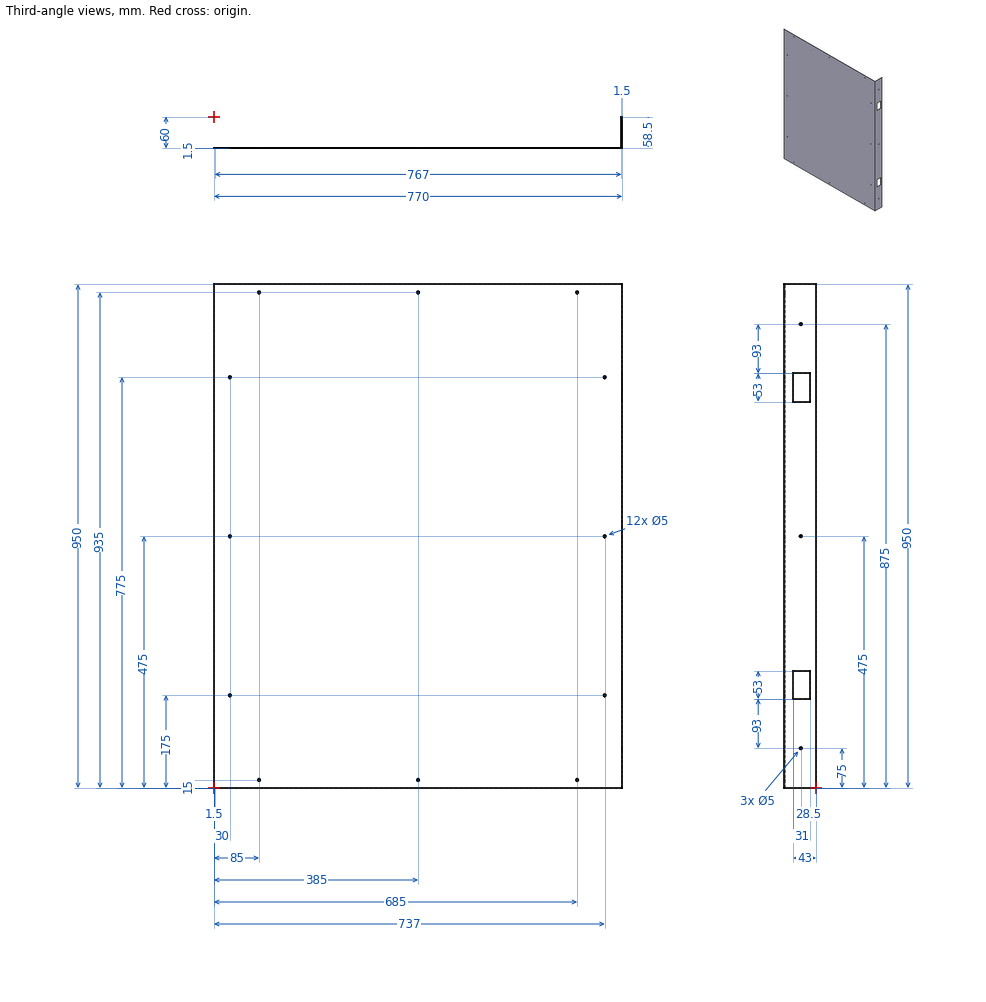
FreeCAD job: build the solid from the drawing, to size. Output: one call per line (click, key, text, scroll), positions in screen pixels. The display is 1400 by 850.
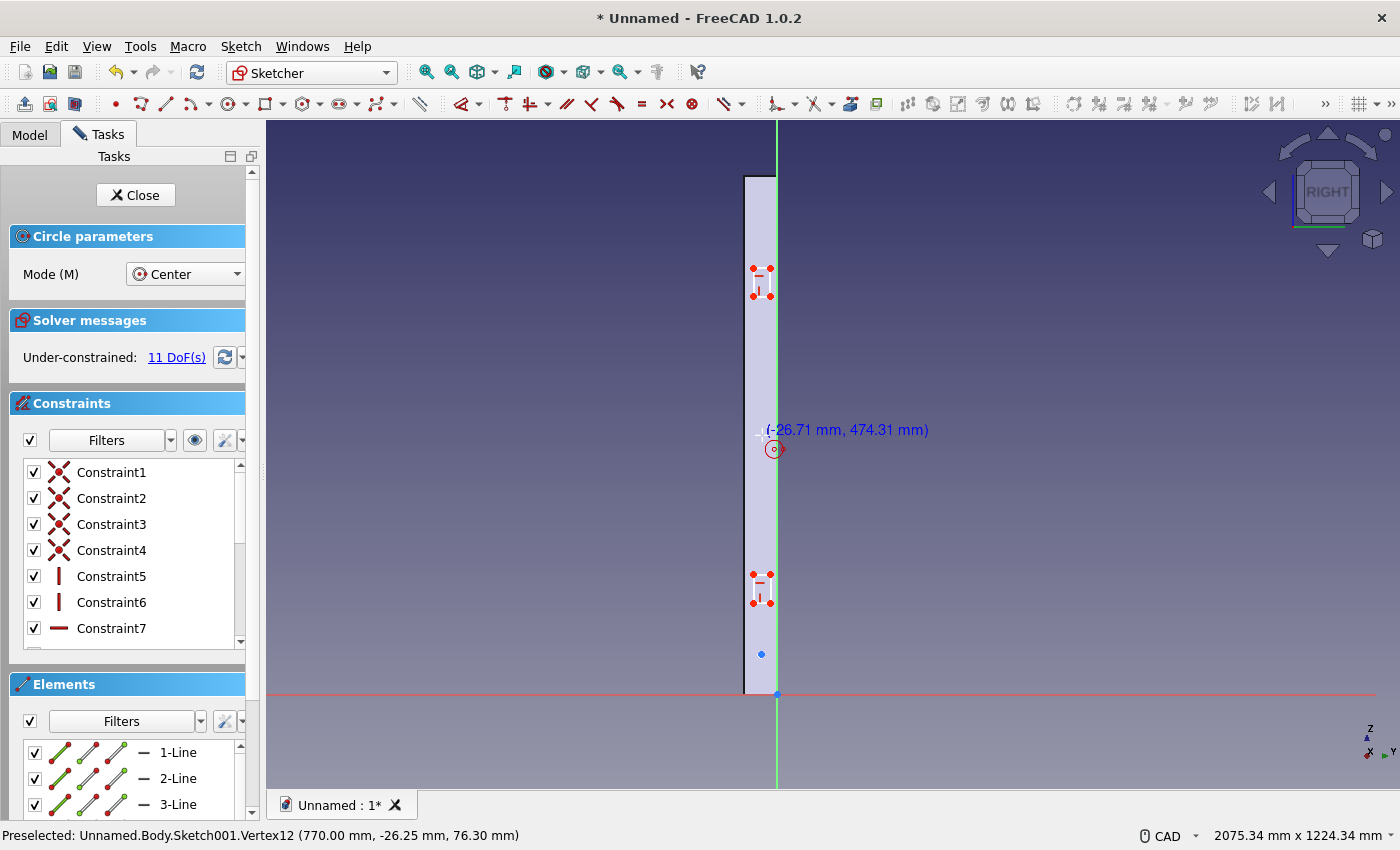
click(761, 435)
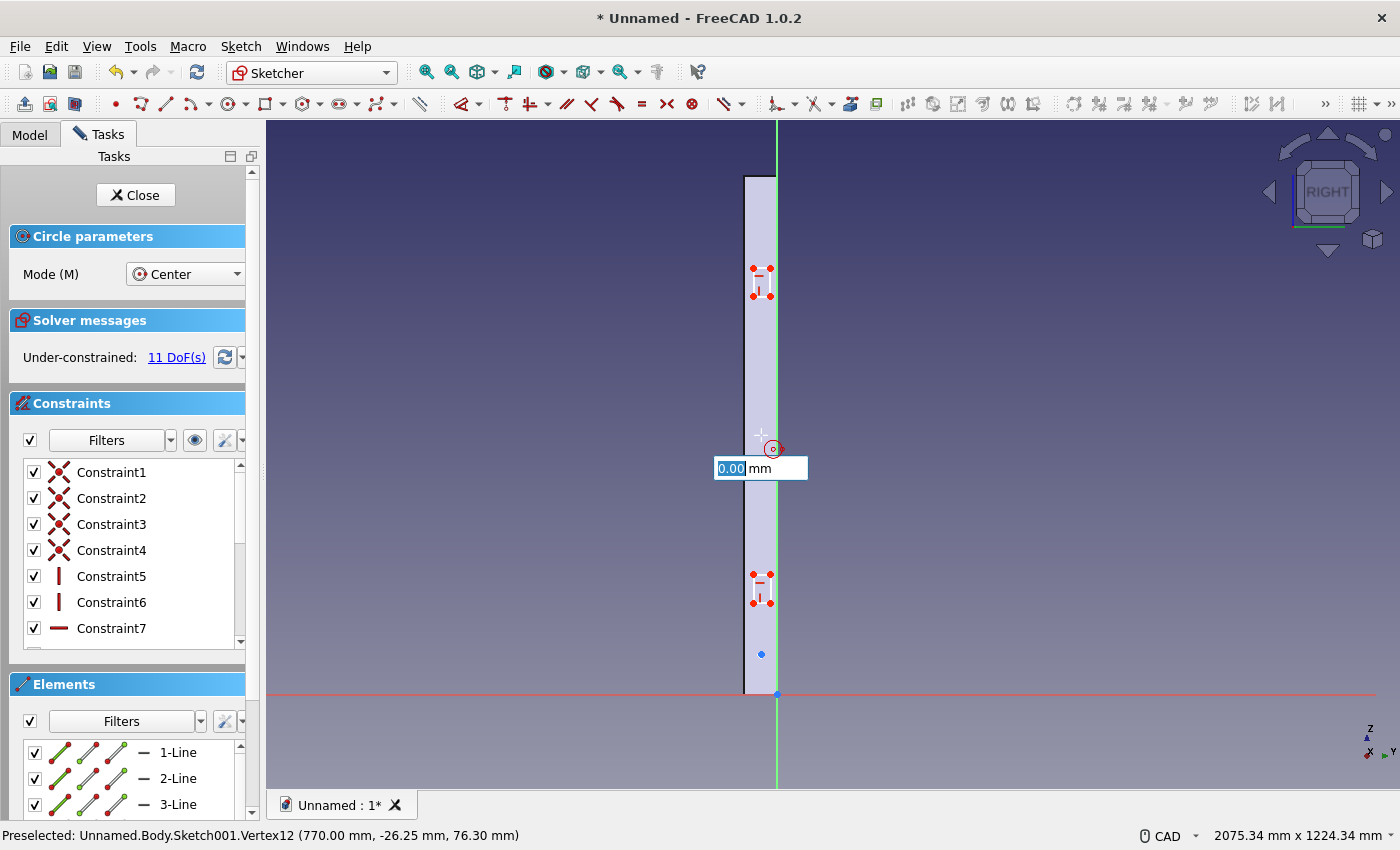
scroll(762, 434, up, 13)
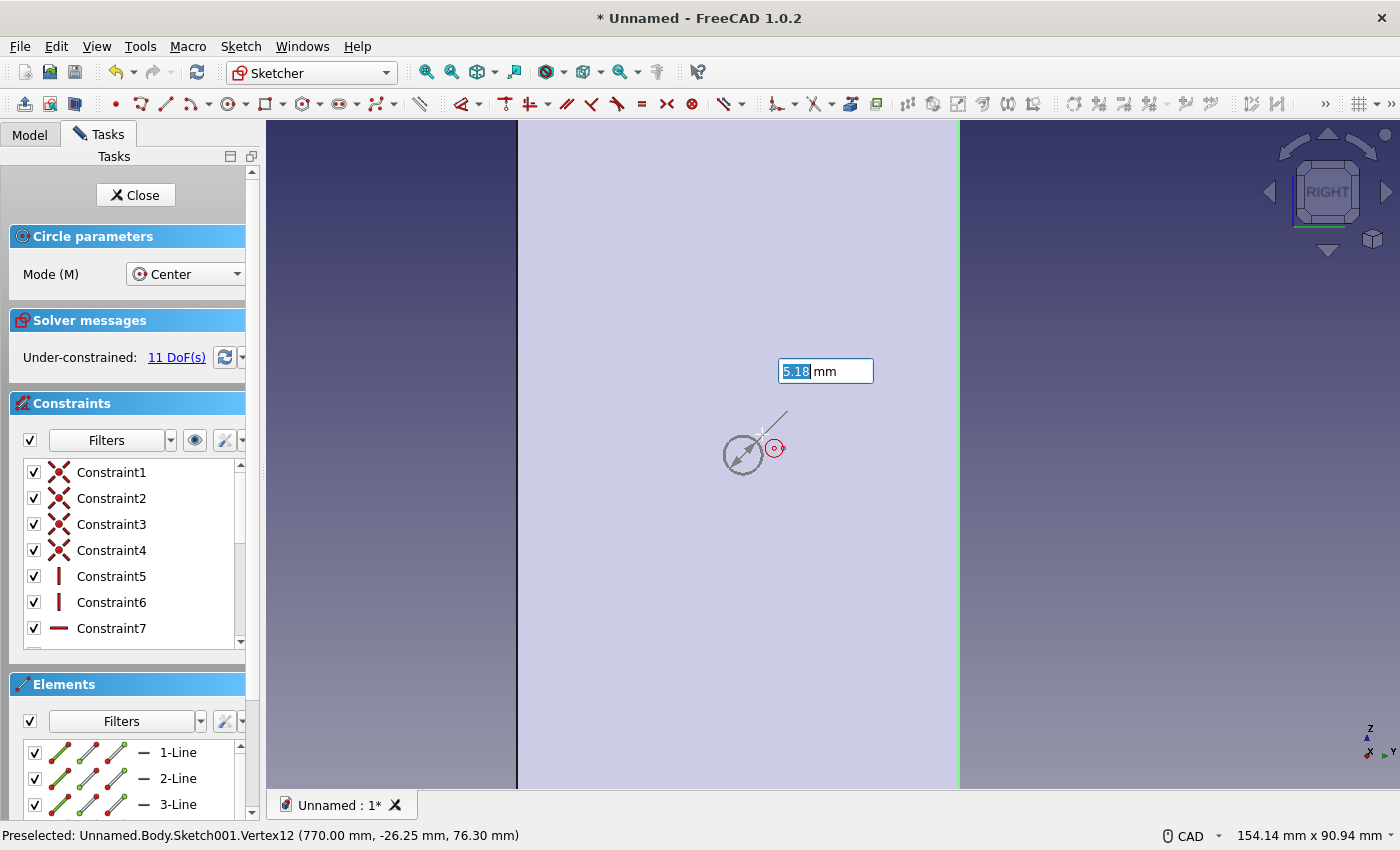
click(762, 430)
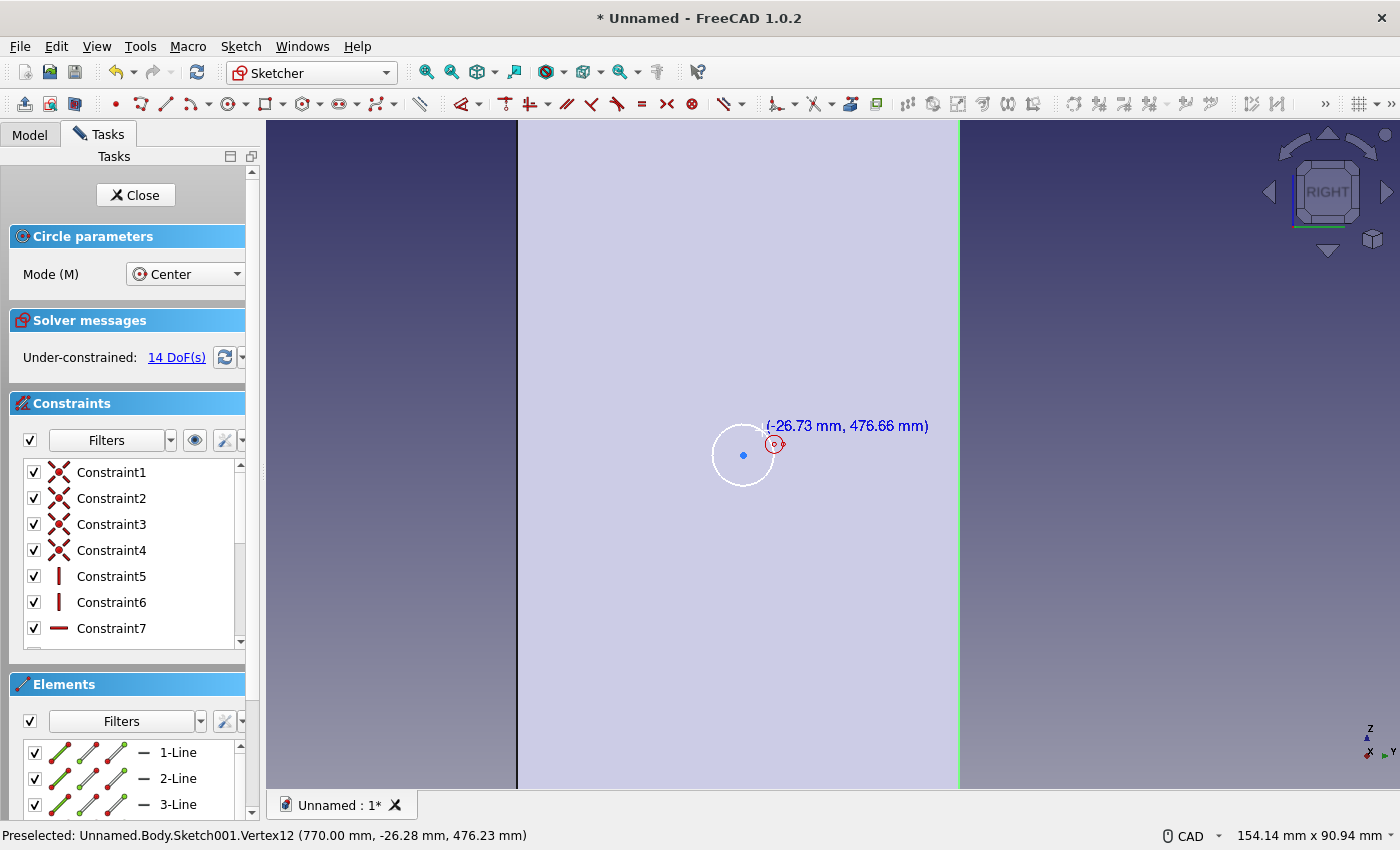
scroll(762, 438, down, 14)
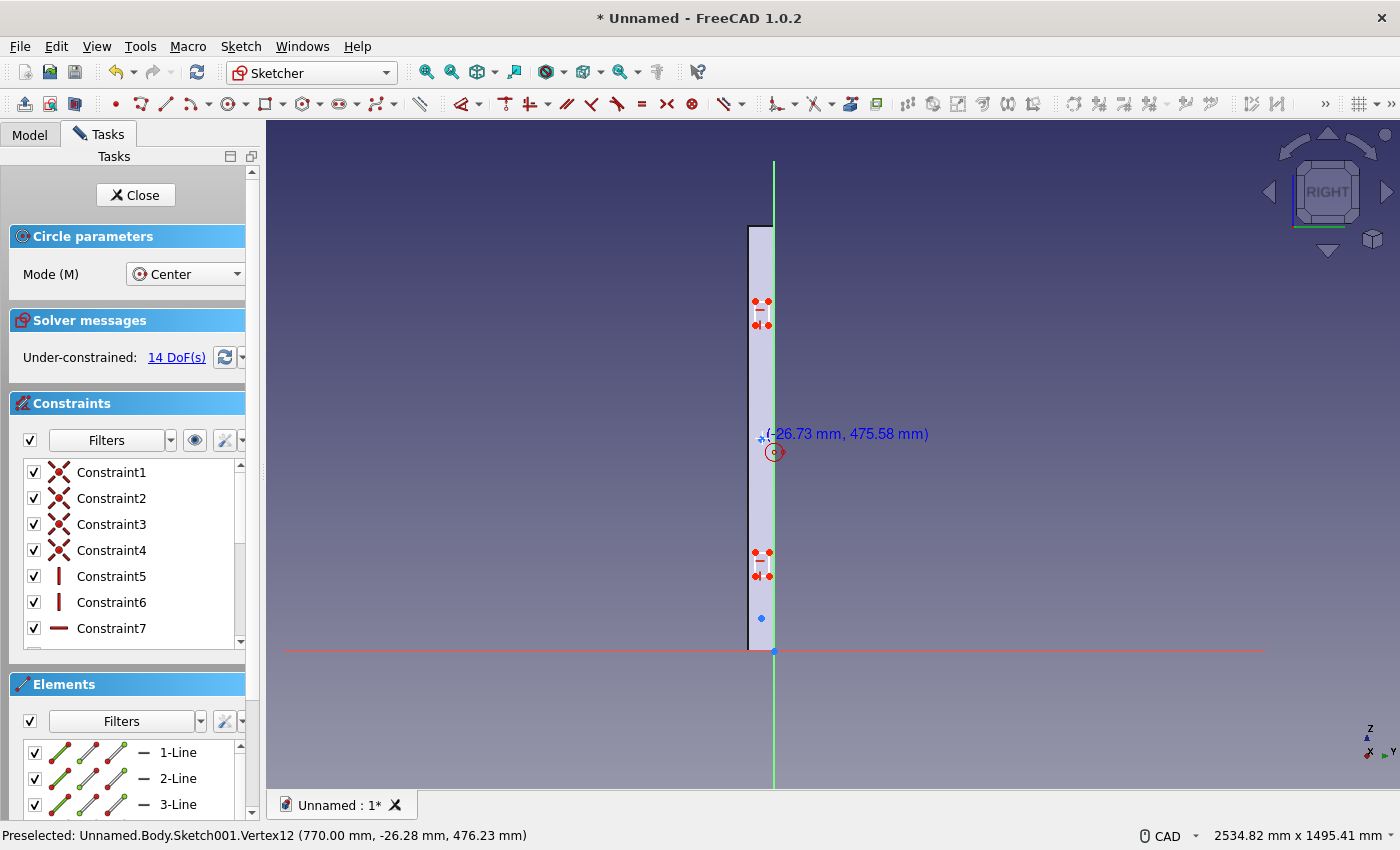
scroll(762, 260, up, 16)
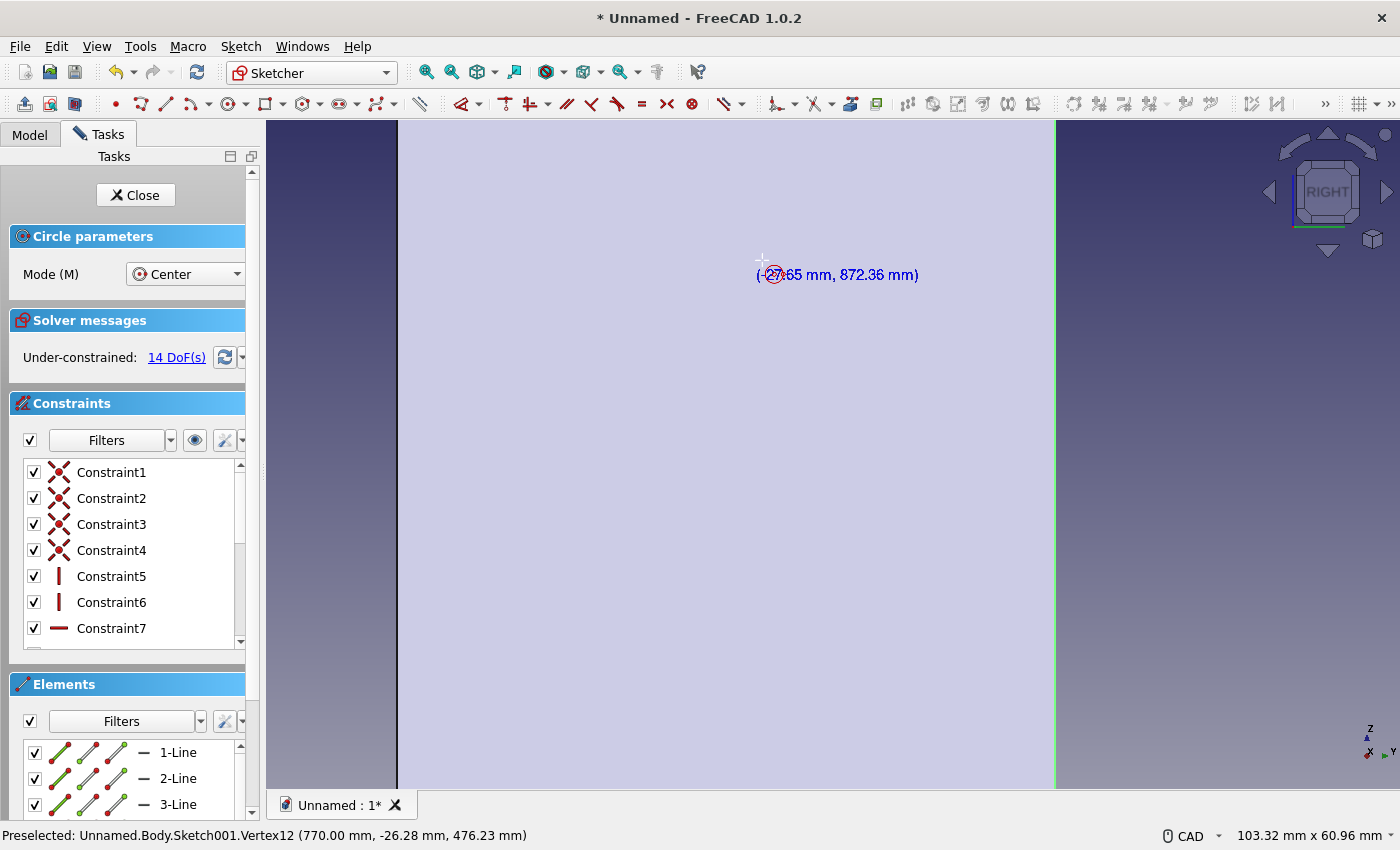
scroll(762, 214, down, 15)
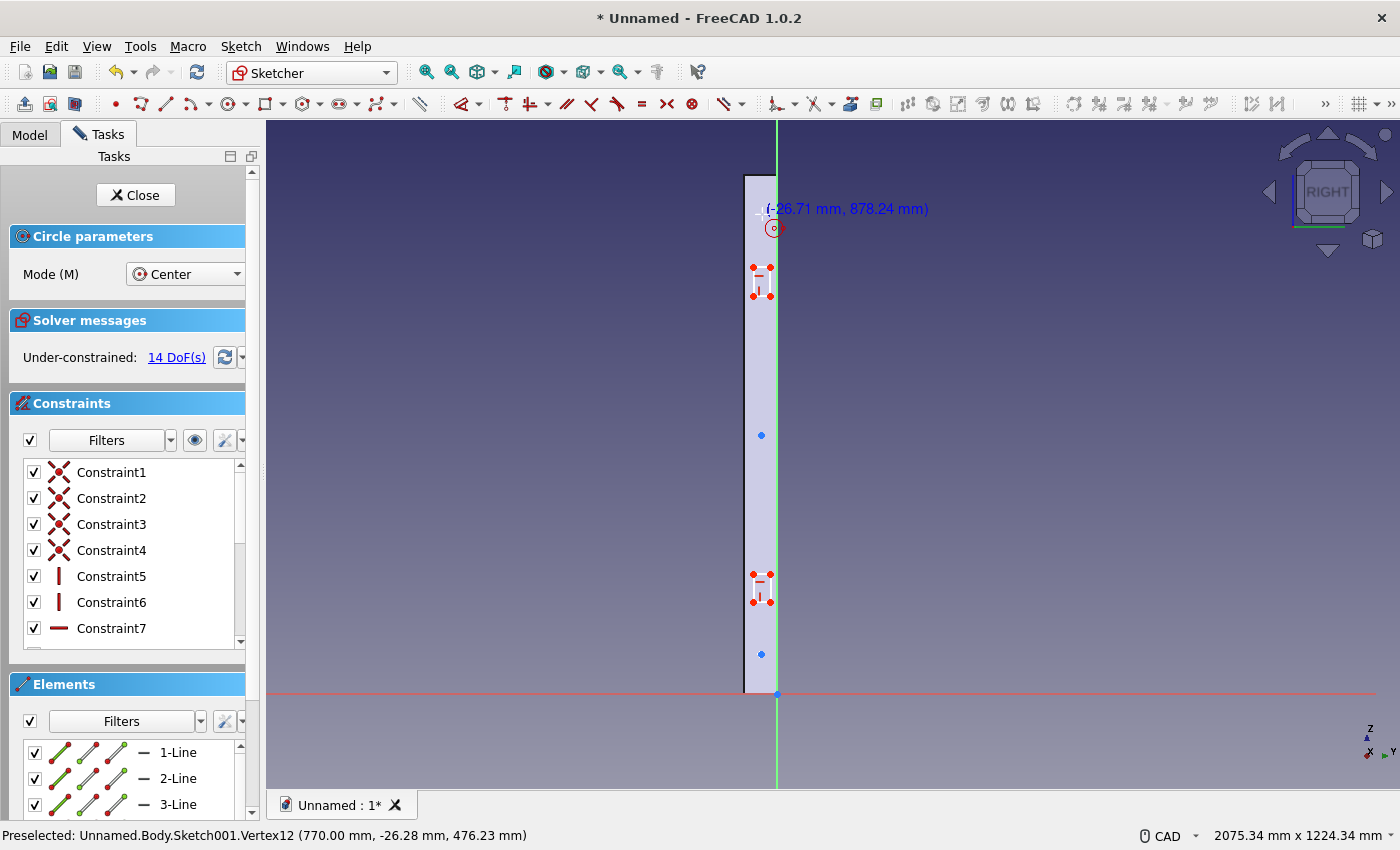
click(761, 216)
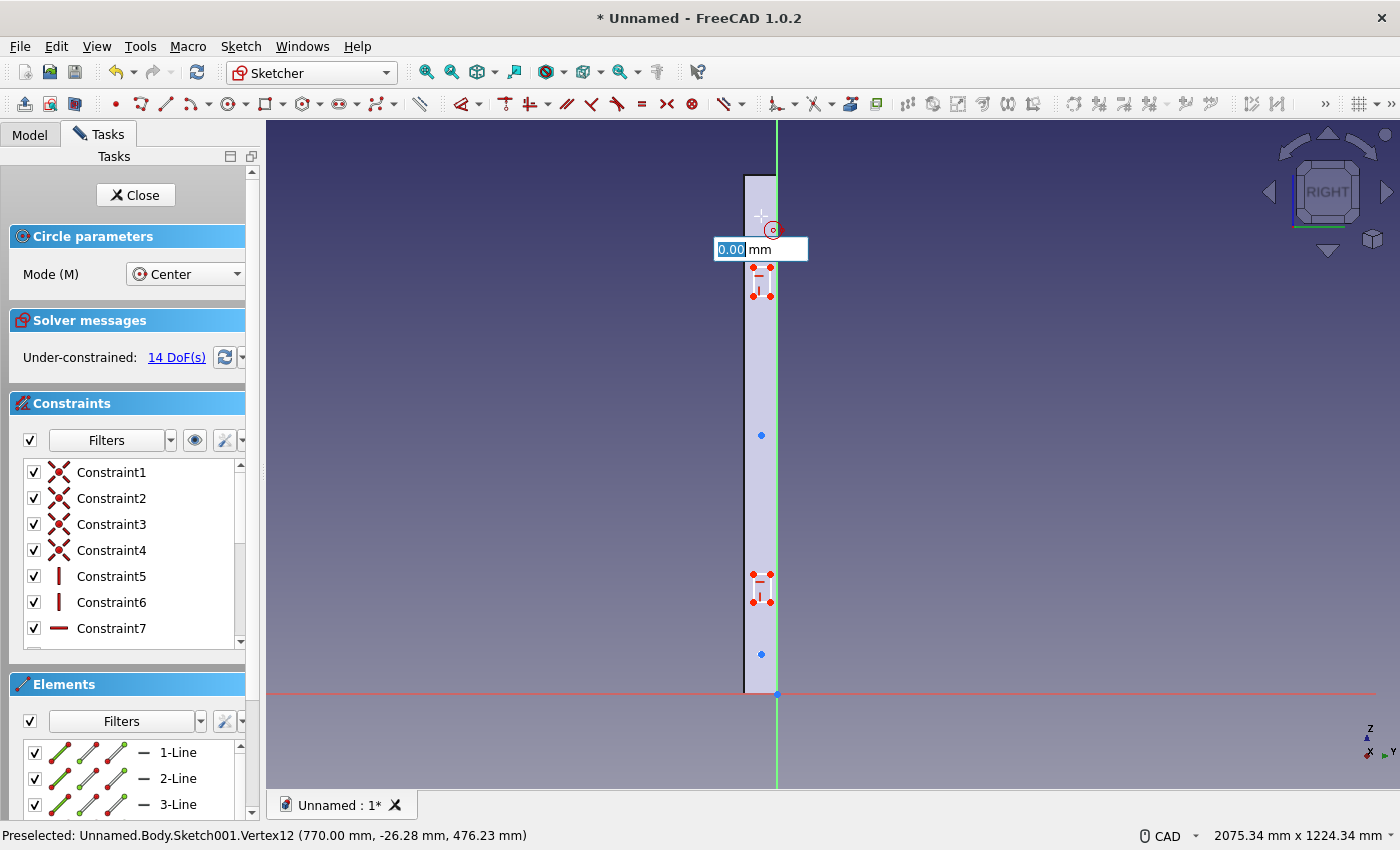
scroll(762, 215, up, 13)